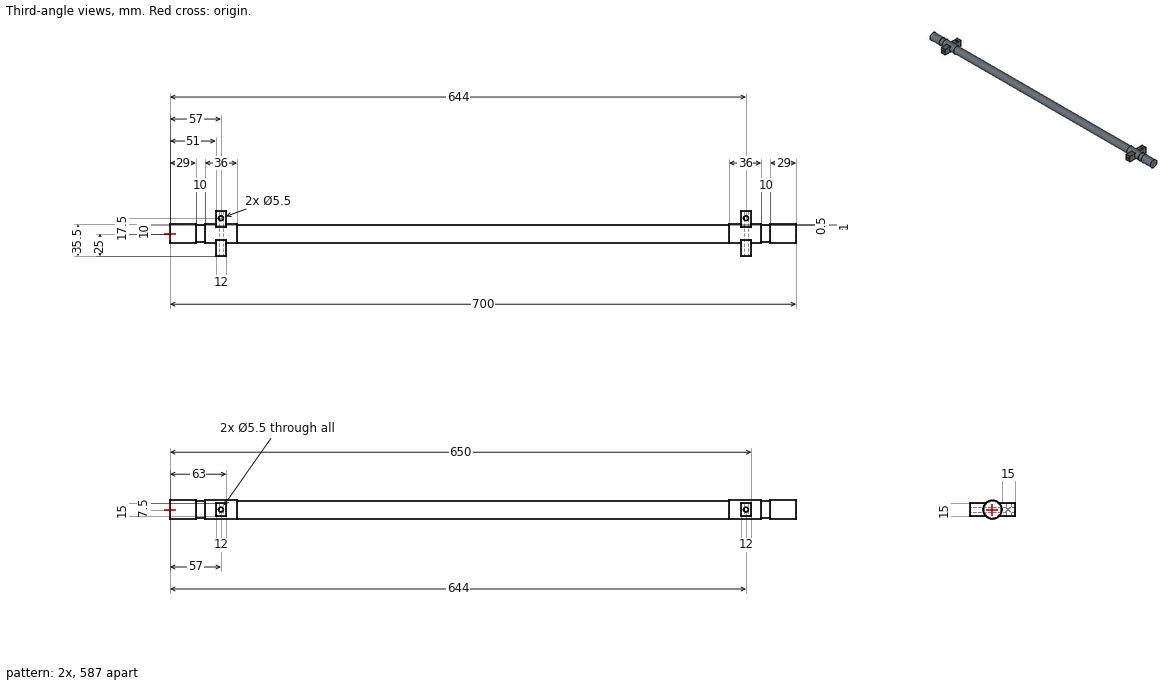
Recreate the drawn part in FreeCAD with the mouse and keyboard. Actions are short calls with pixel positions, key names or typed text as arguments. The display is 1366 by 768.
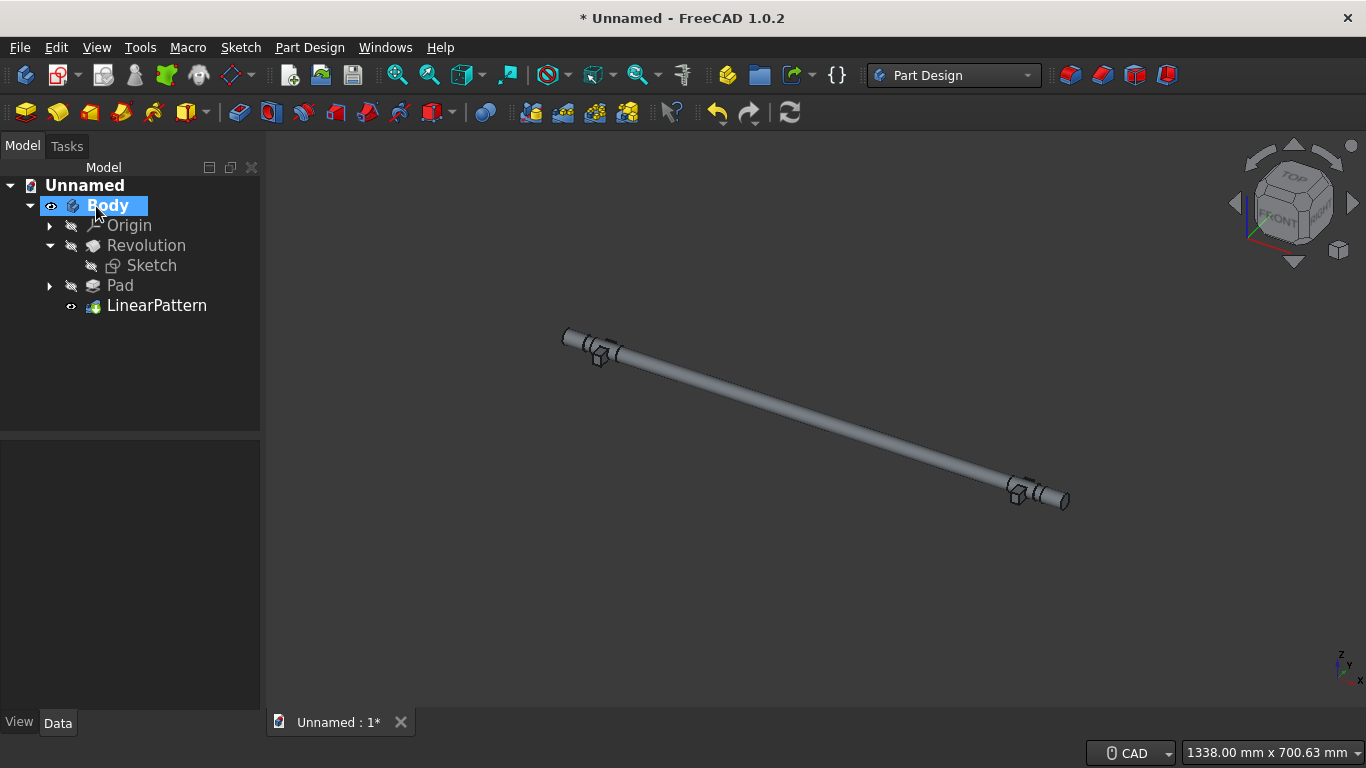
key(4)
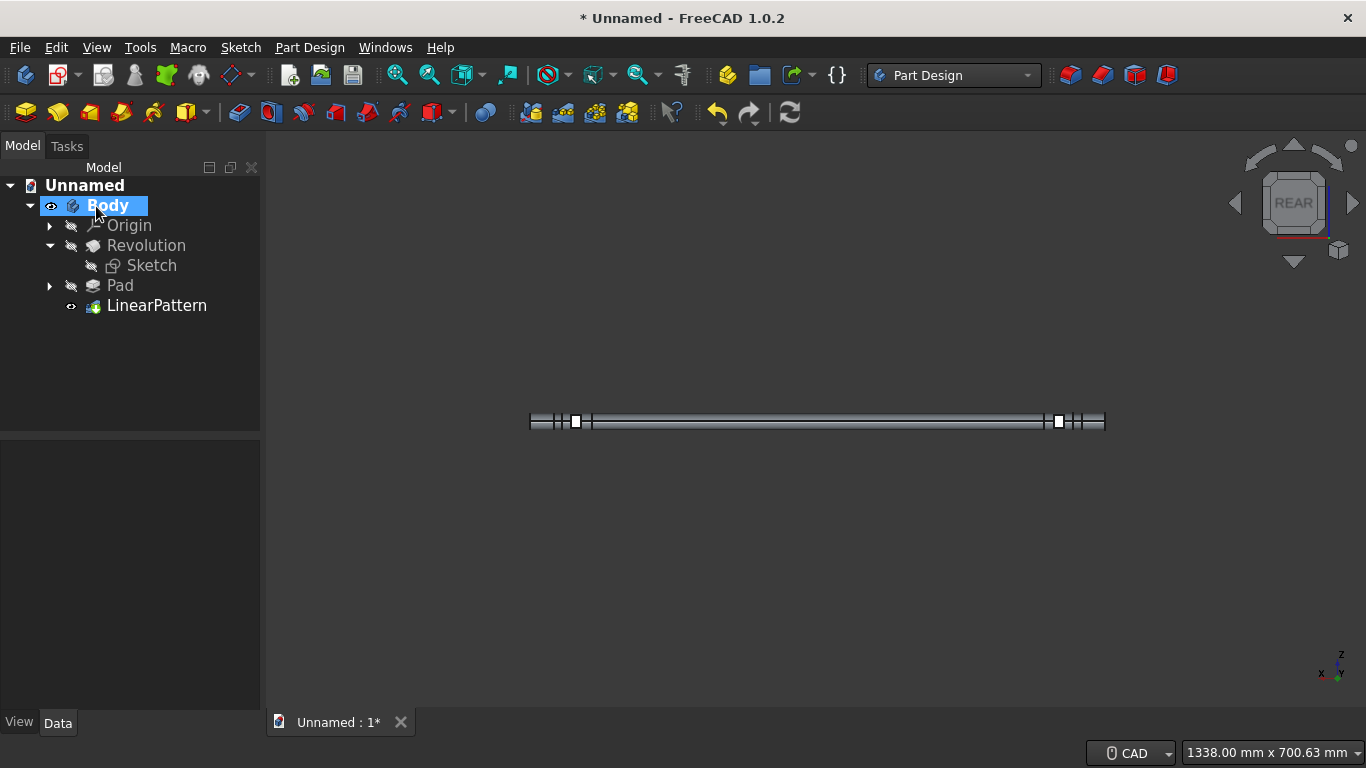
scroll(576, 420, up, 5)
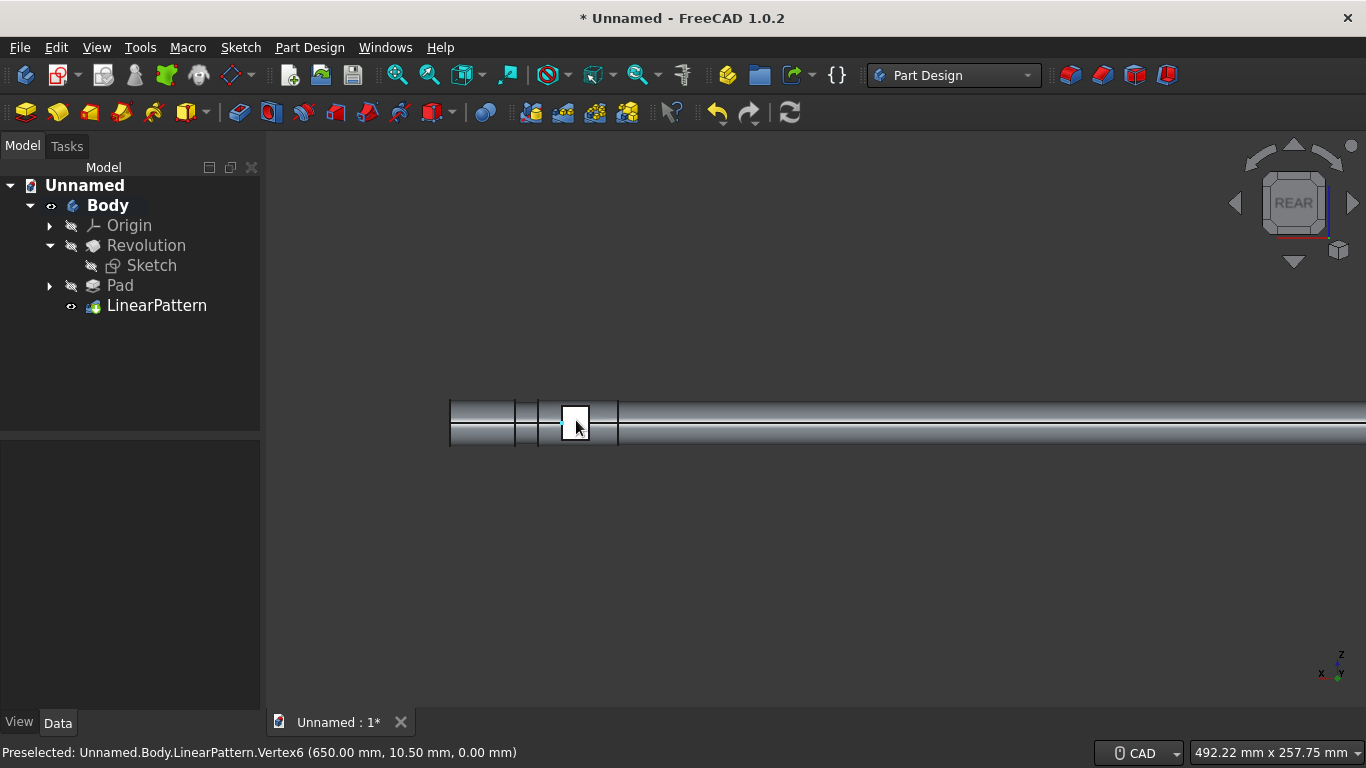
click(576, 422)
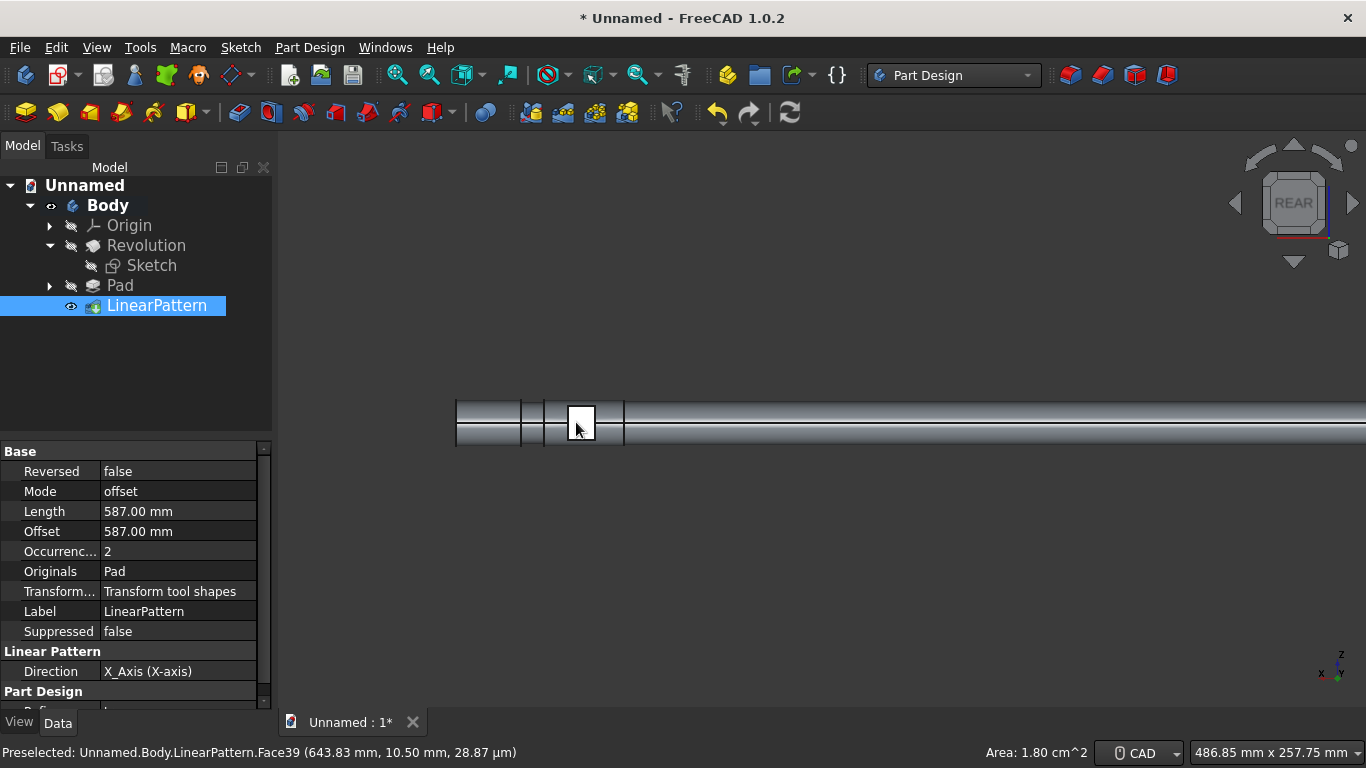
click(58, 76)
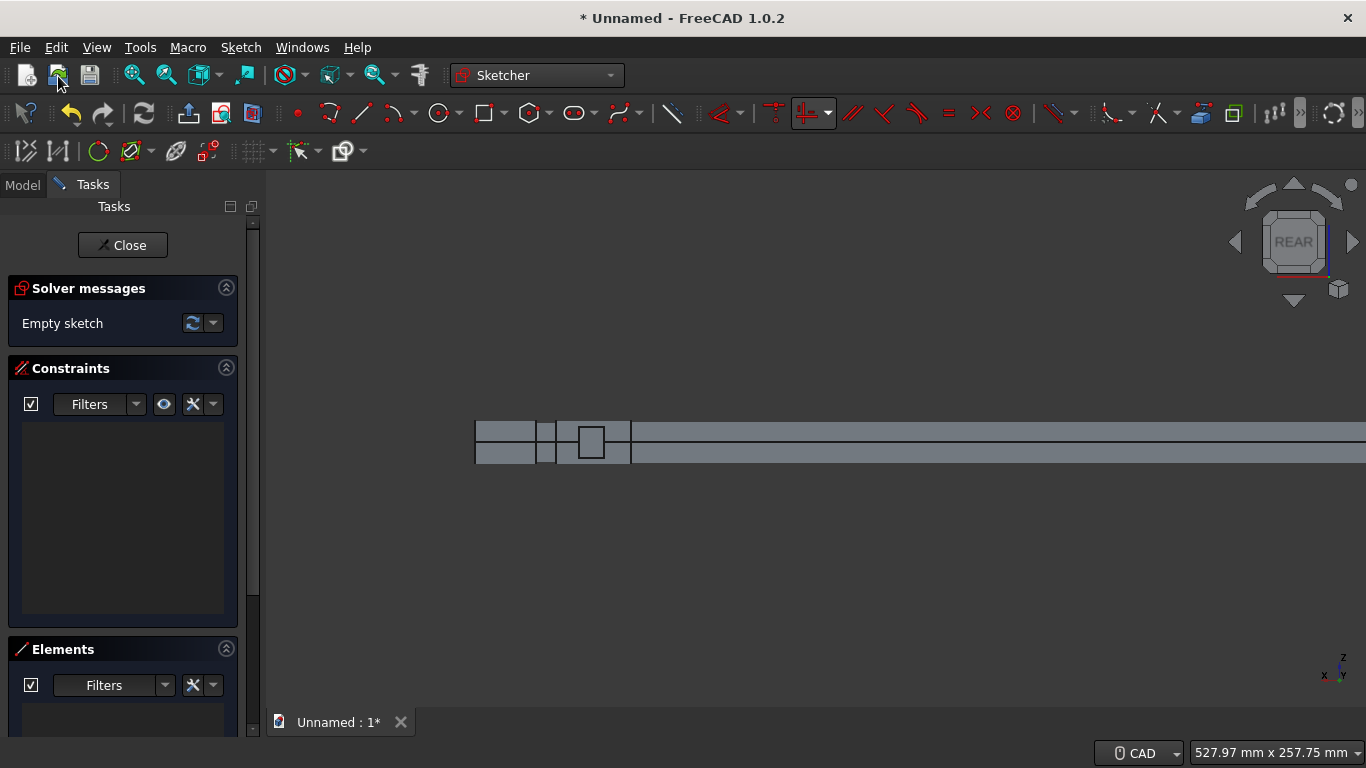
scroll(332, 435, down, 4)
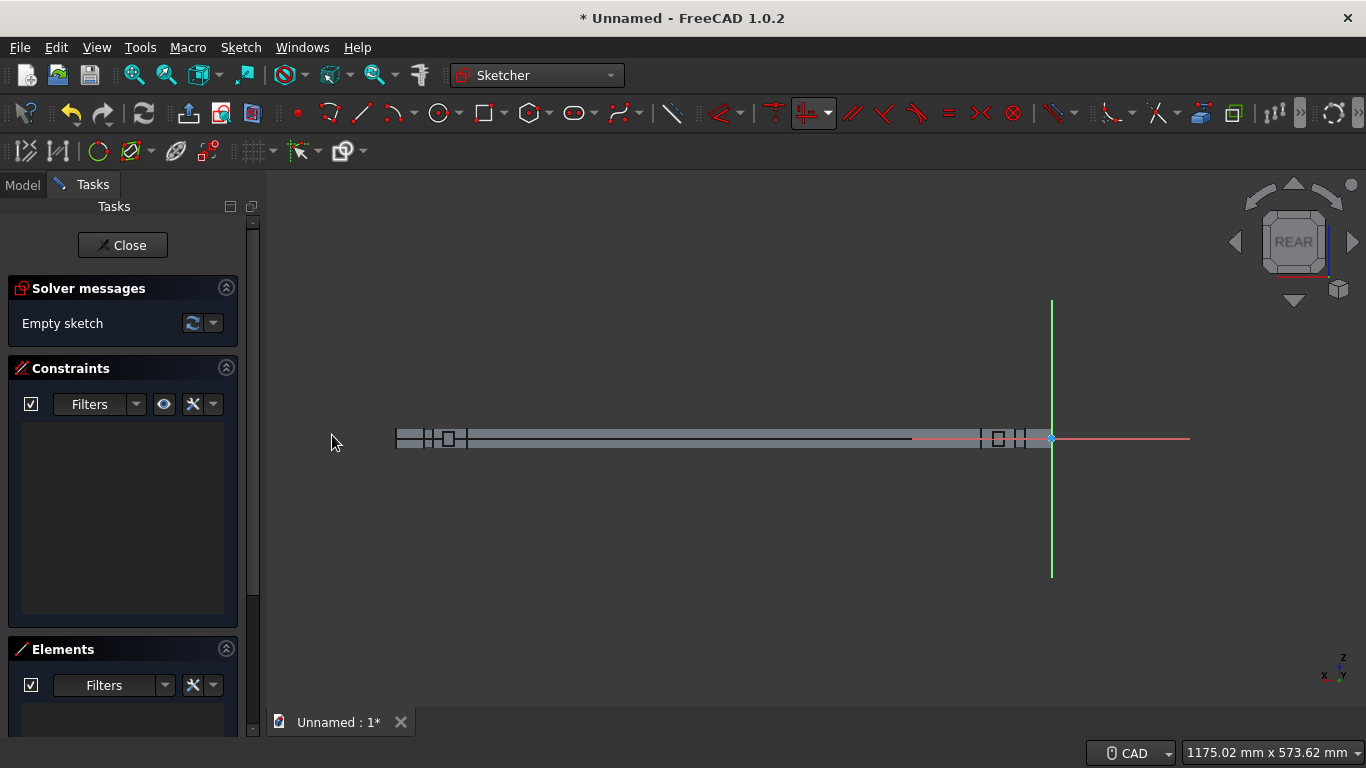
click(484, 114)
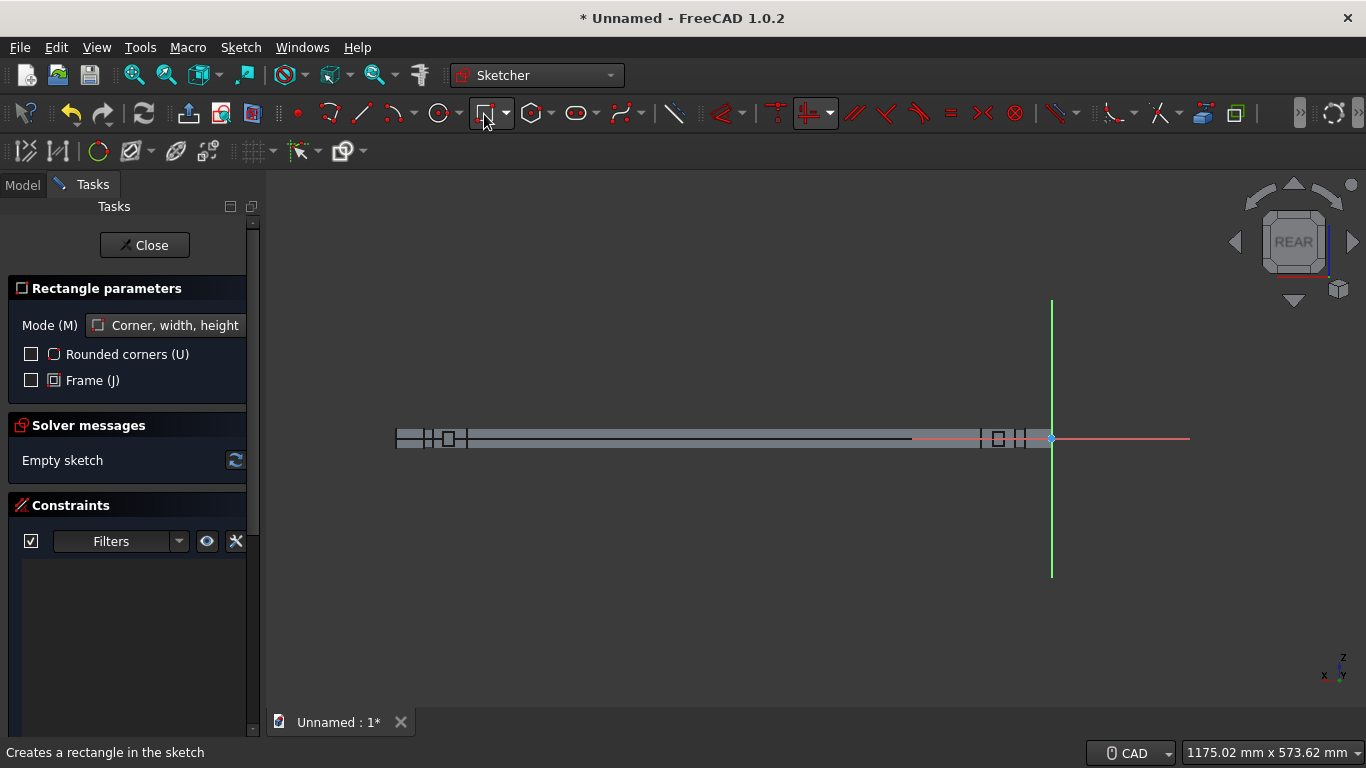
scroll(993, 432, up, 5)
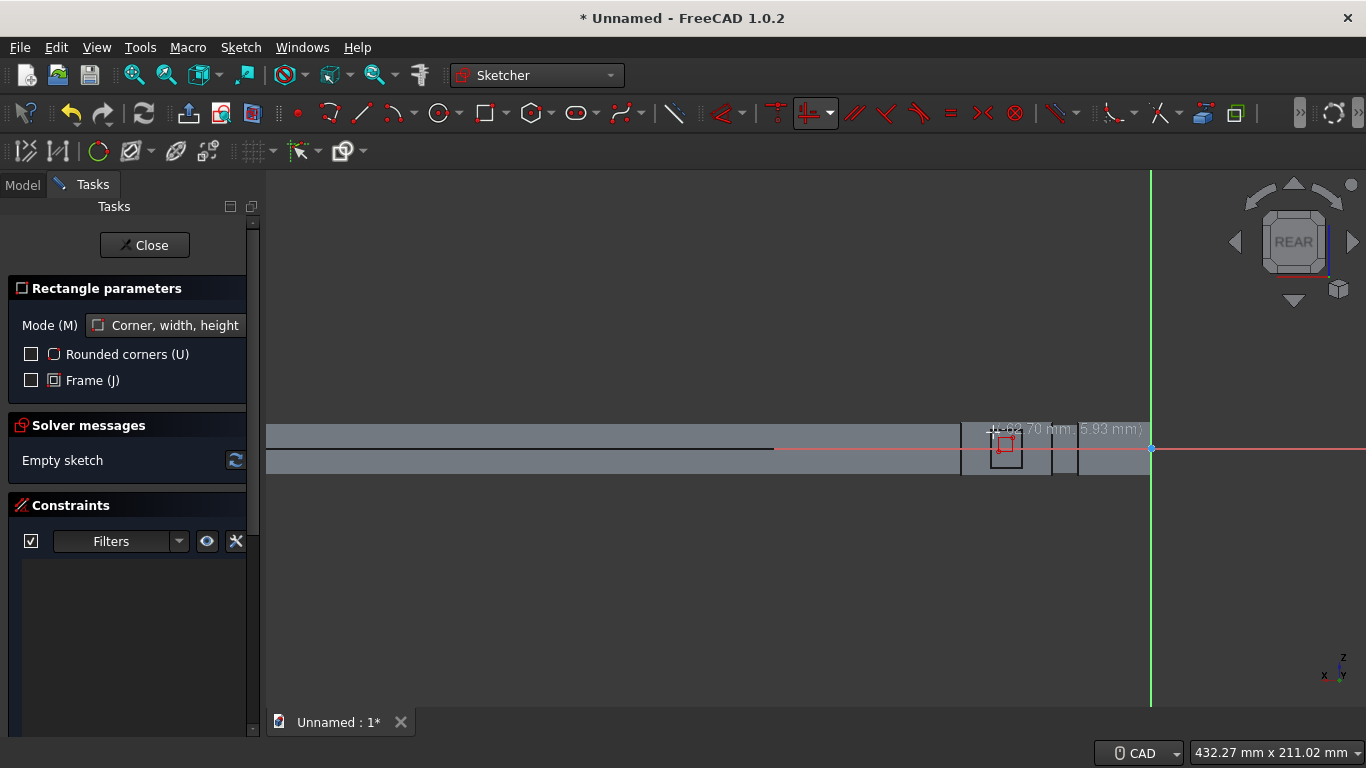
click(991, 430)
click(1022, 468)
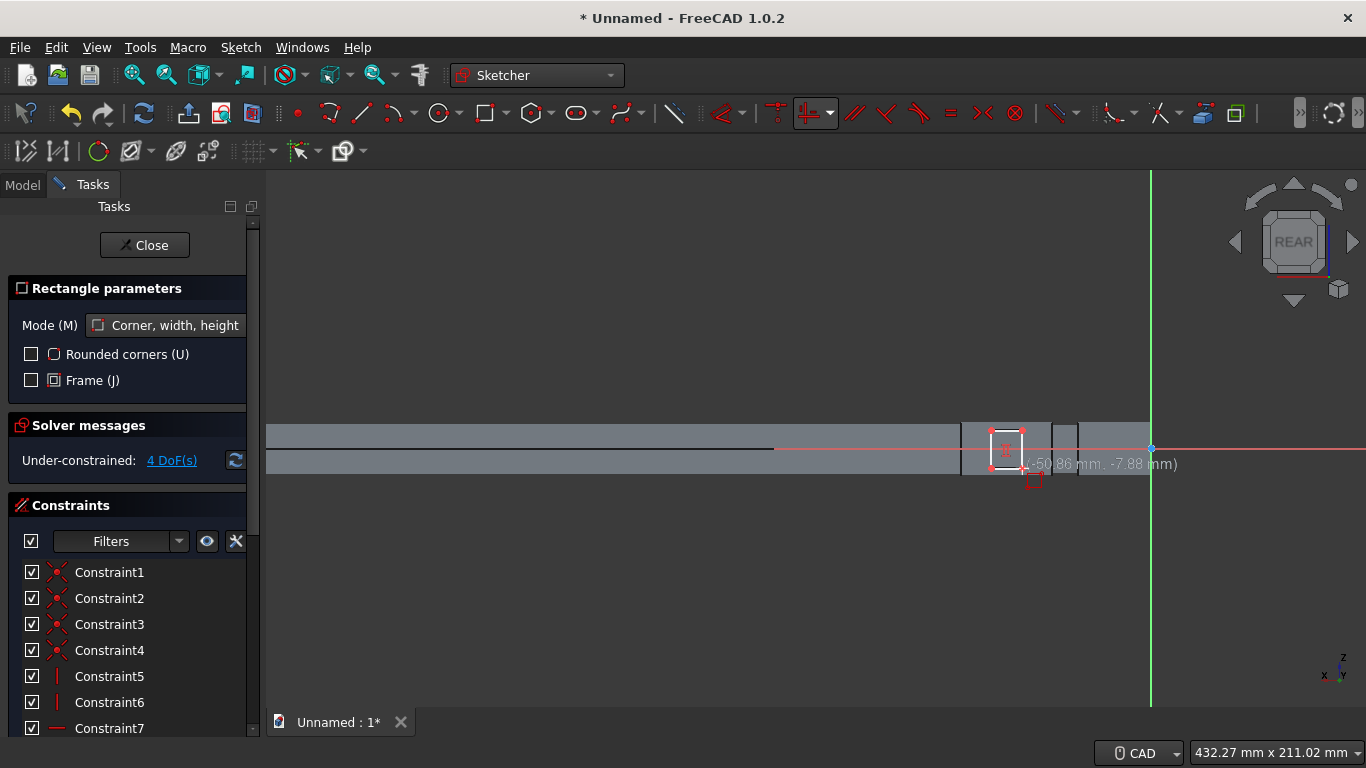
scroll(994, 432, down, 5)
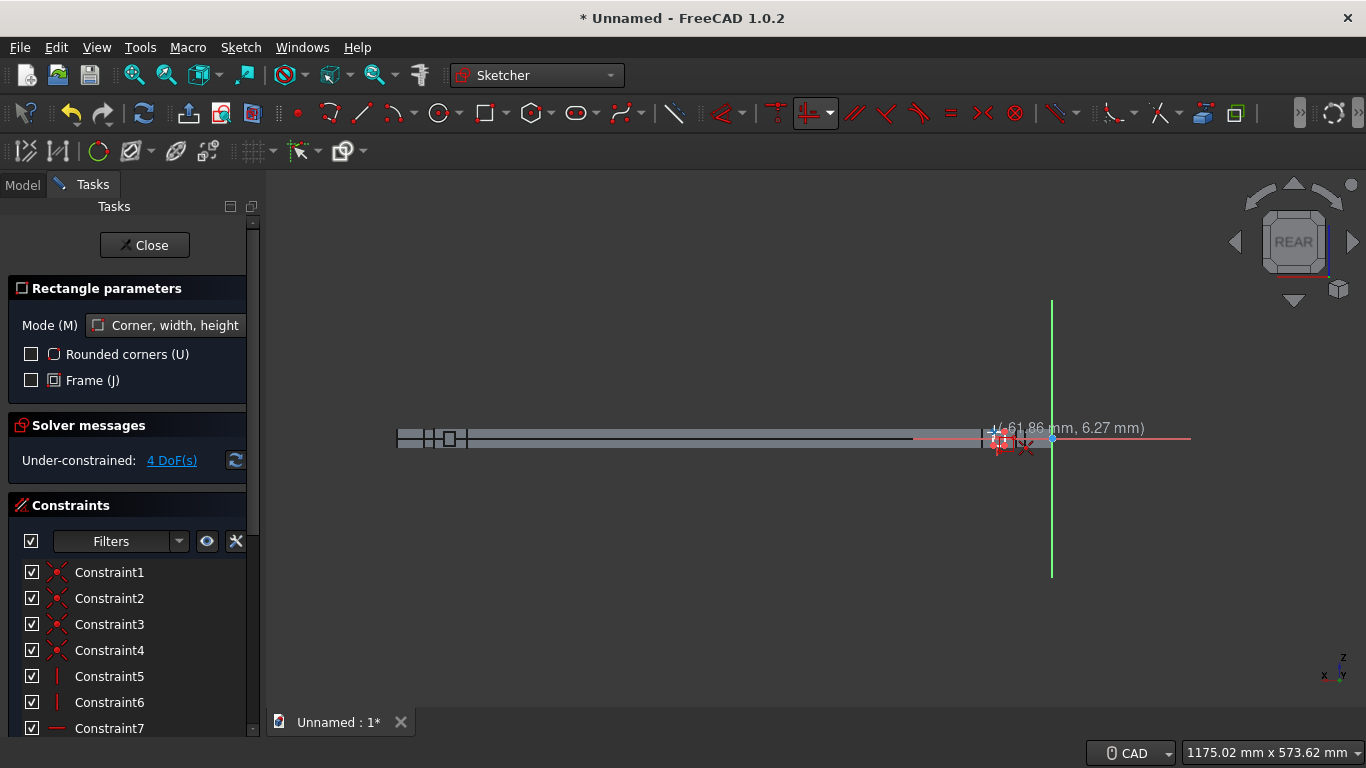
scroll(444, 432, up, 5)